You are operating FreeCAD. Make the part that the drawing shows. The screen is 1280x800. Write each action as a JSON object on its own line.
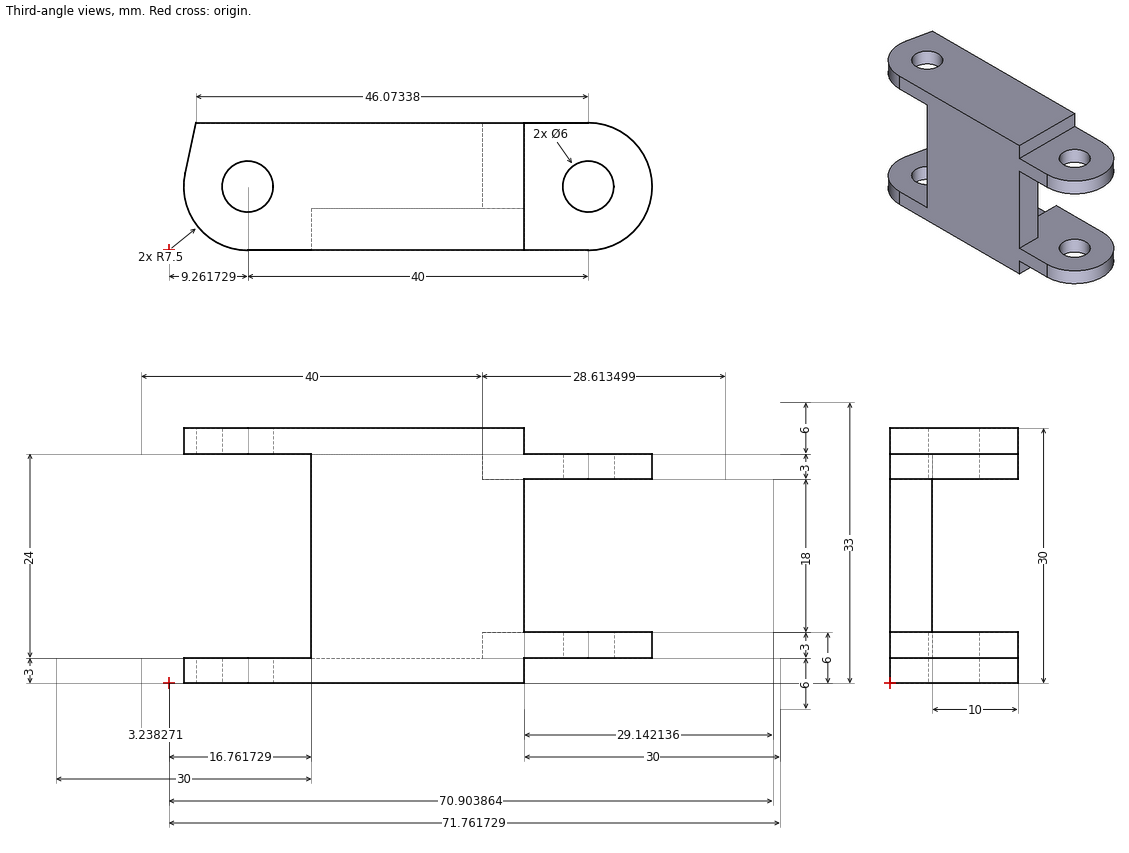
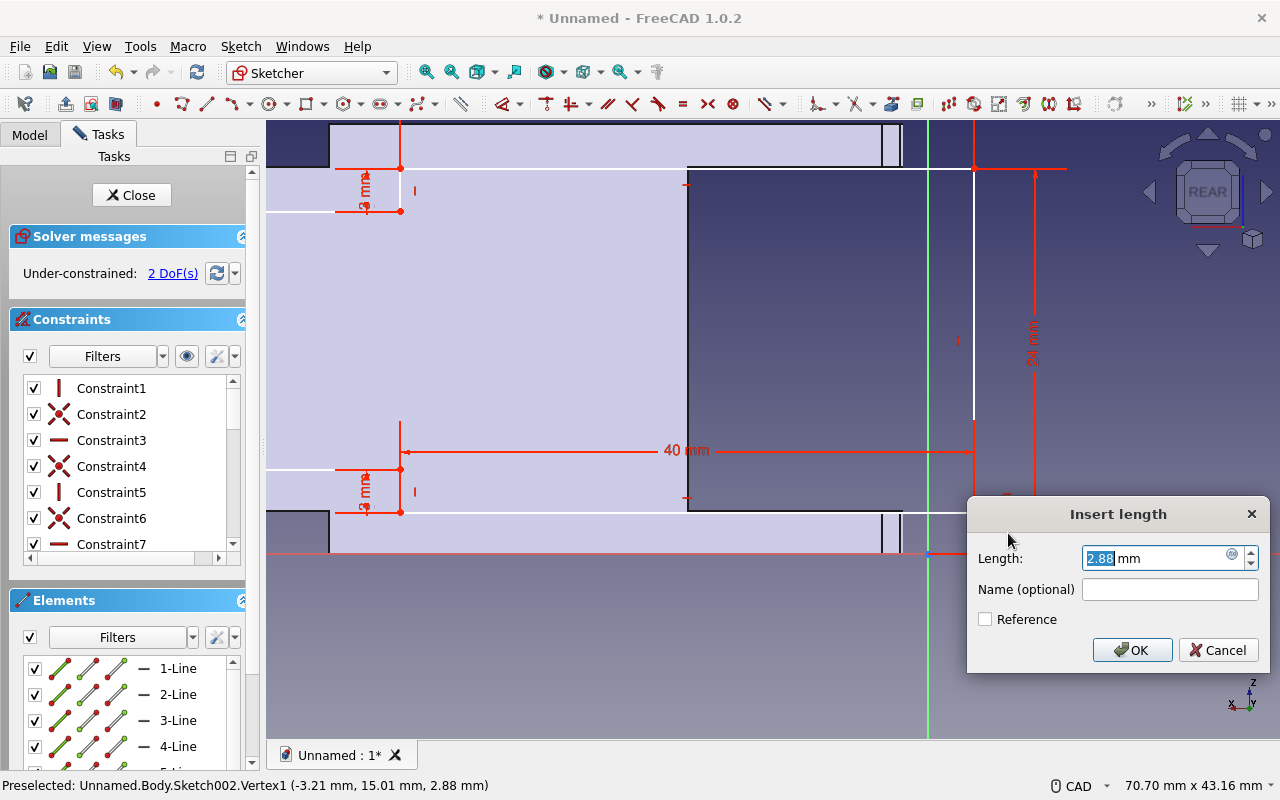
{"action": "type", "text": "3"}
{"action": "key", "text": "Return"}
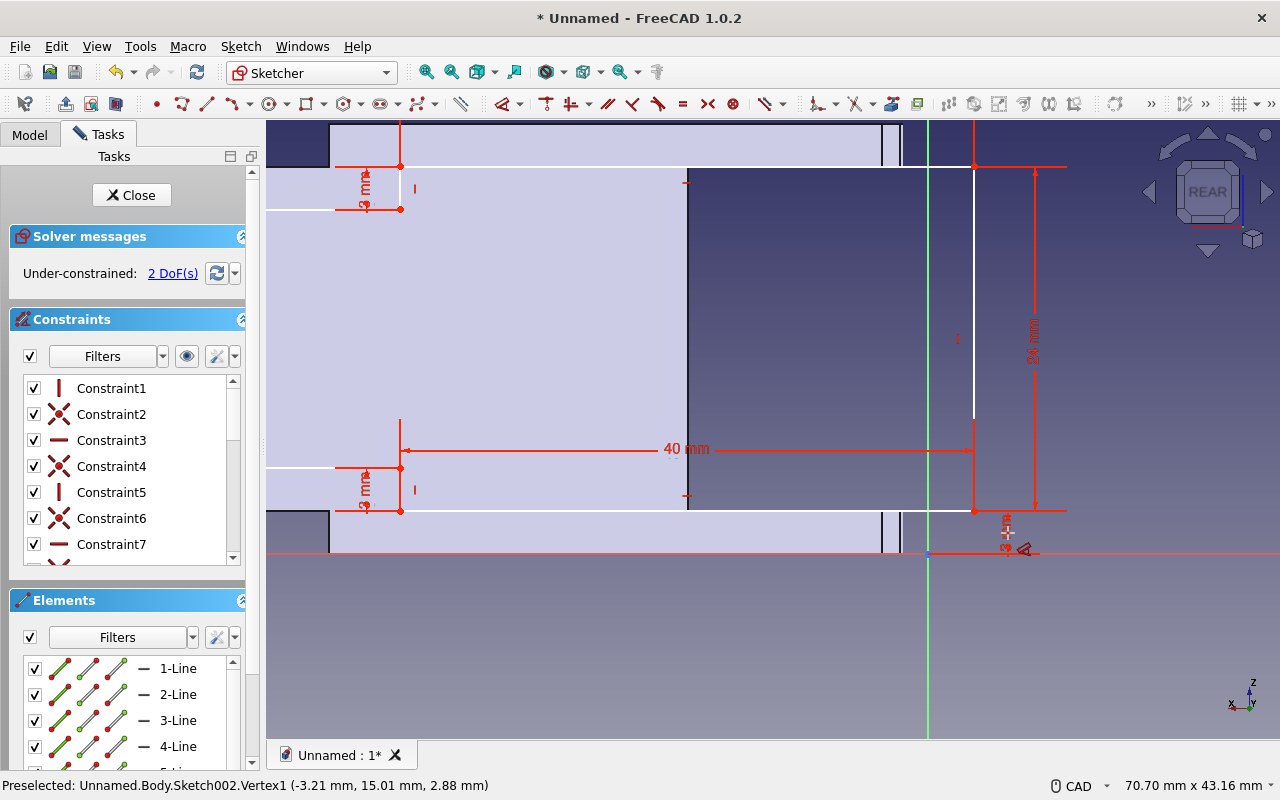
{"action": "left_click", "coordinate": [319, 210]}
{"action": "left_click", "coordinate": [347, 244]}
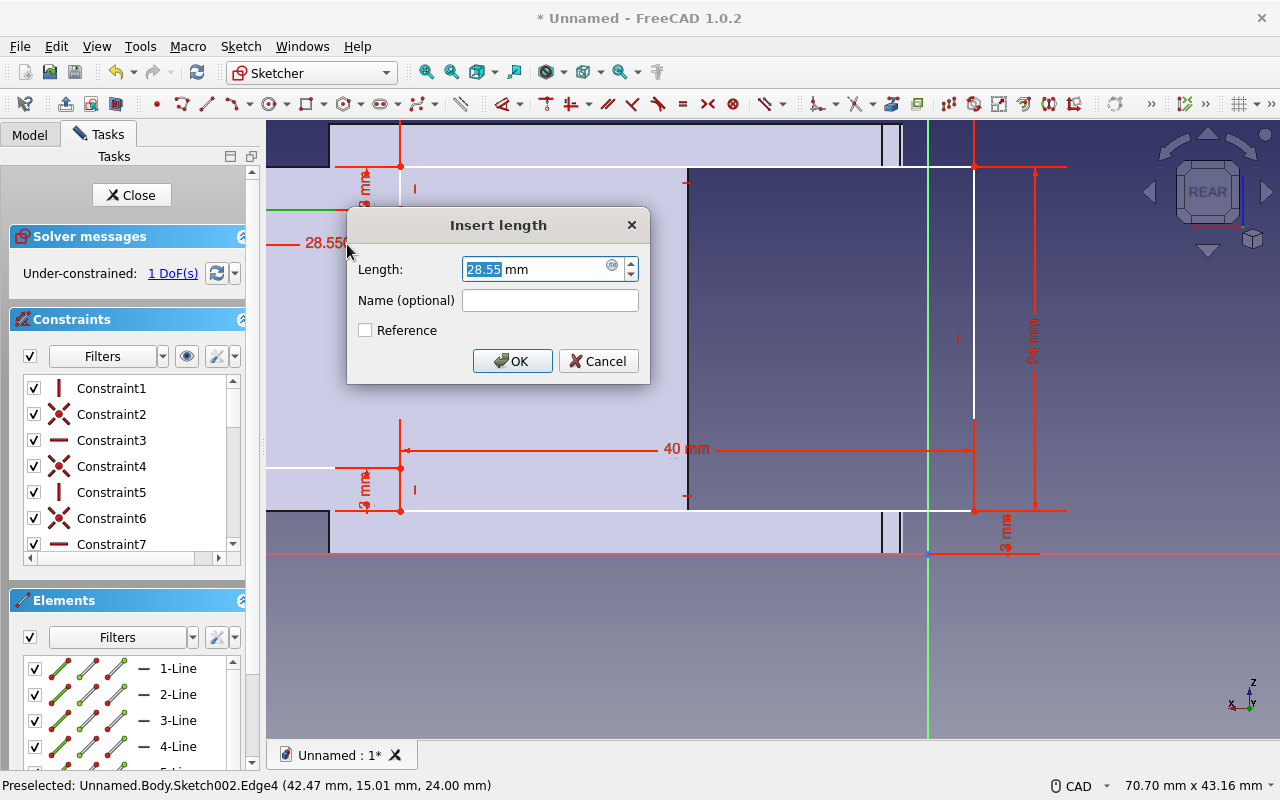
{"action": "type", "text": "28.613499"}
{"action": "key", "text": "Return"}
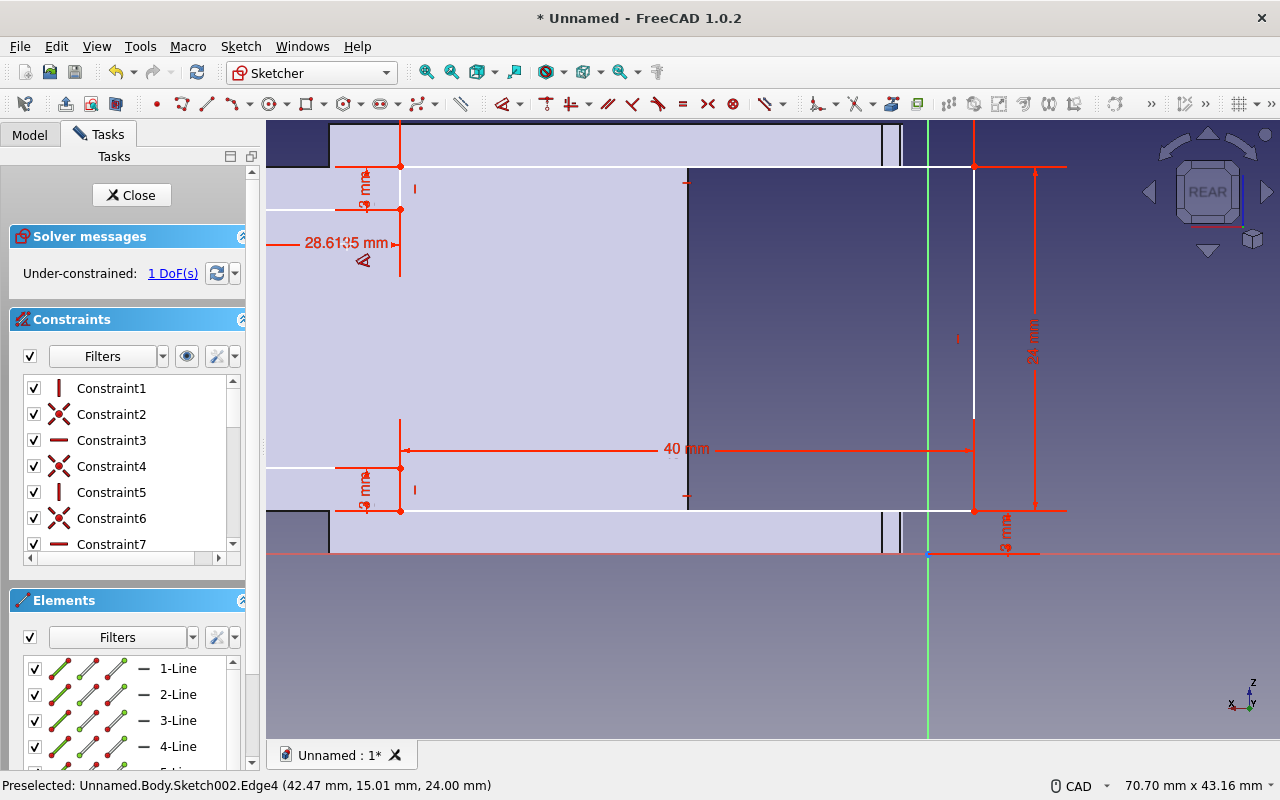
{"action": "left_click", "coordinate": [974, 511]}
{"action": "left_click", "coordinate": [951, 588]}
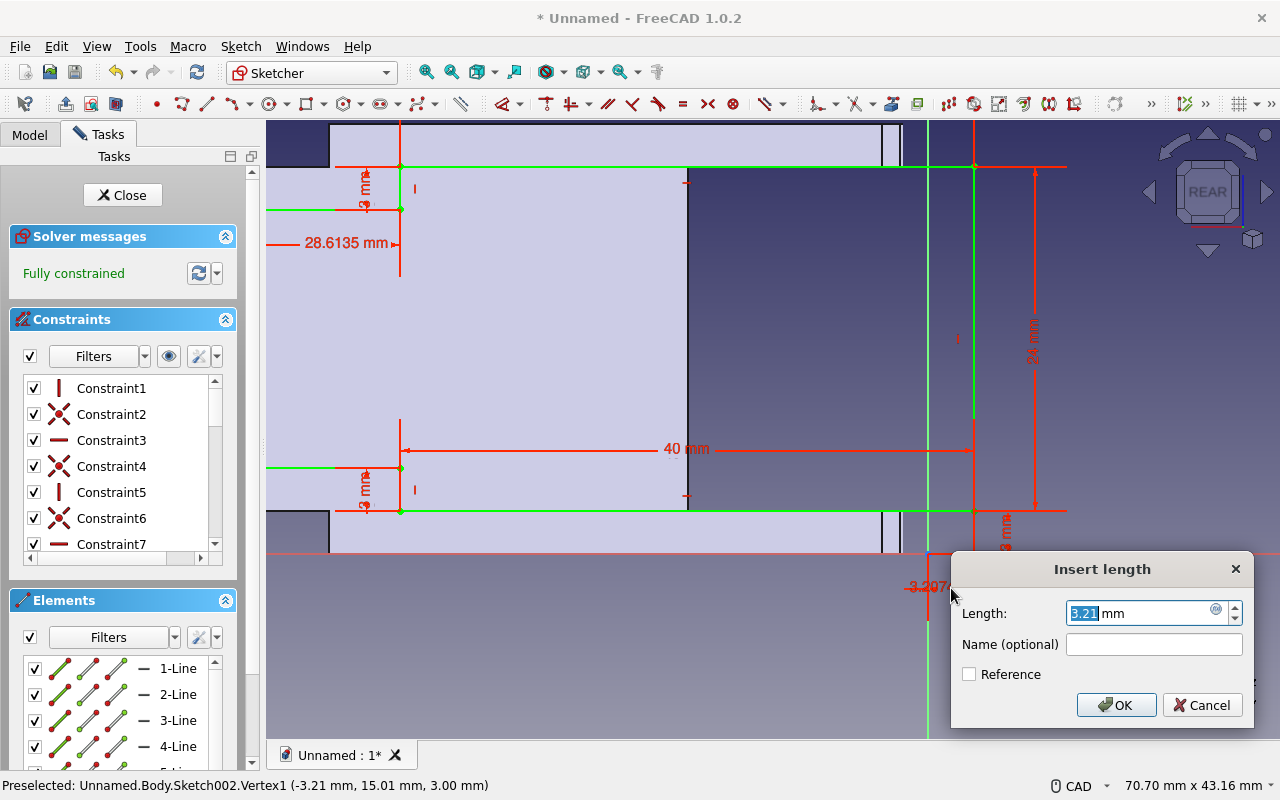
{"action": "type", "text": "3.238271"}
{"action": "key", "text": "Return"}
{"action": "key", "text": "Escape"}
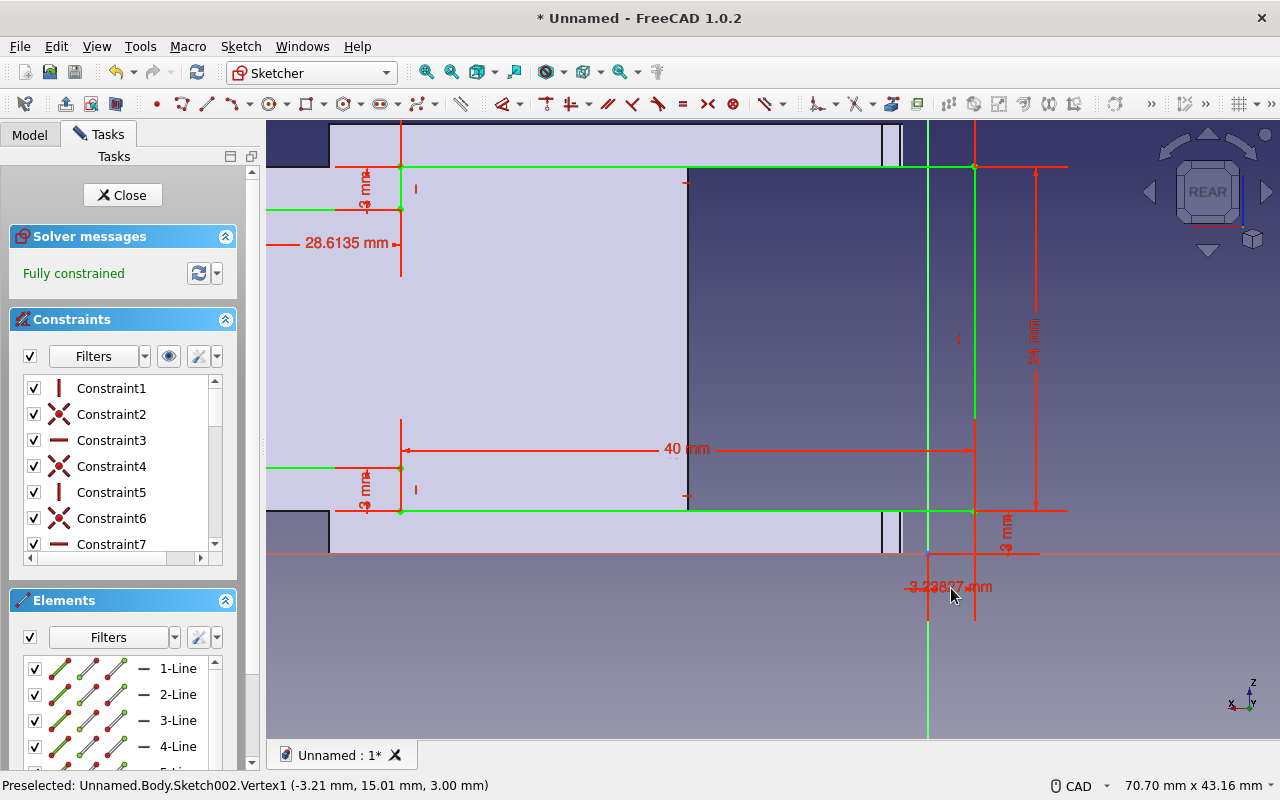
{"action": "left_click", "coordinate": [123, 195]}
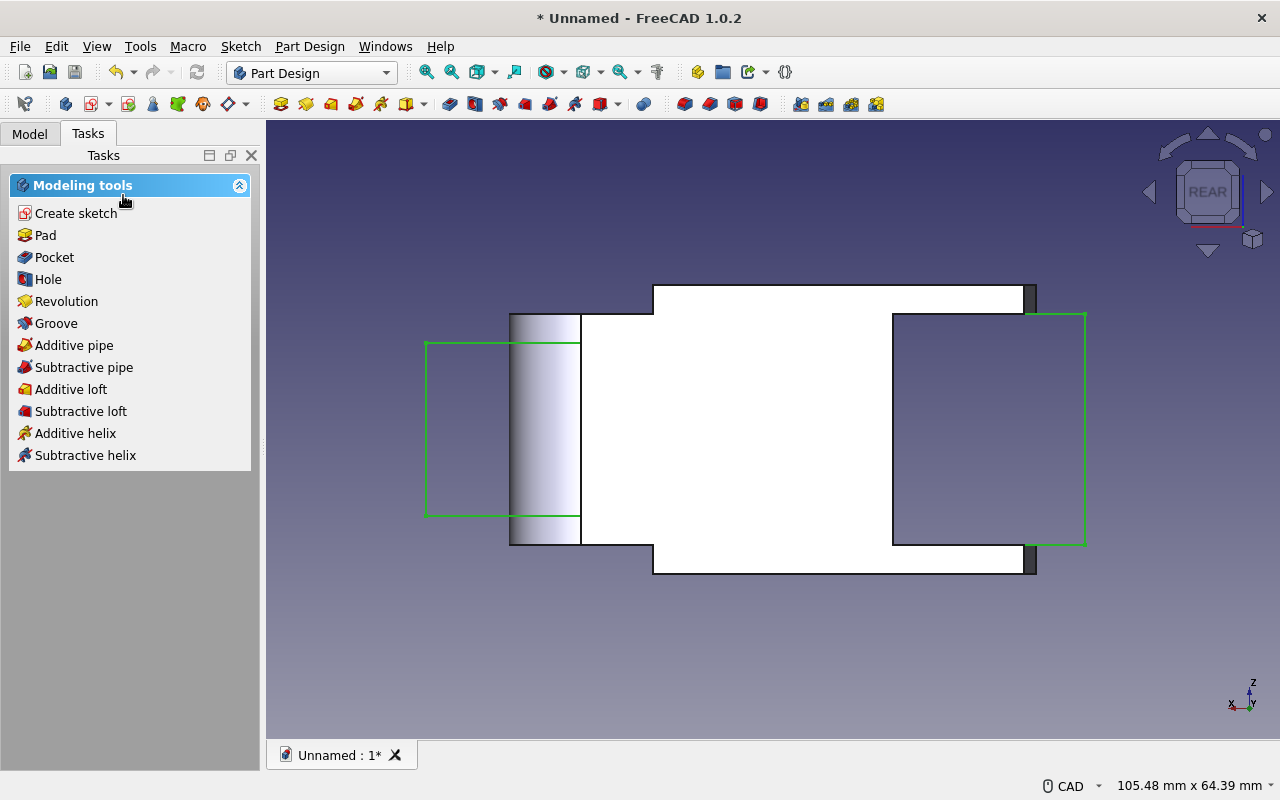
{"action": "left_click", "coordinate": [450, 104]}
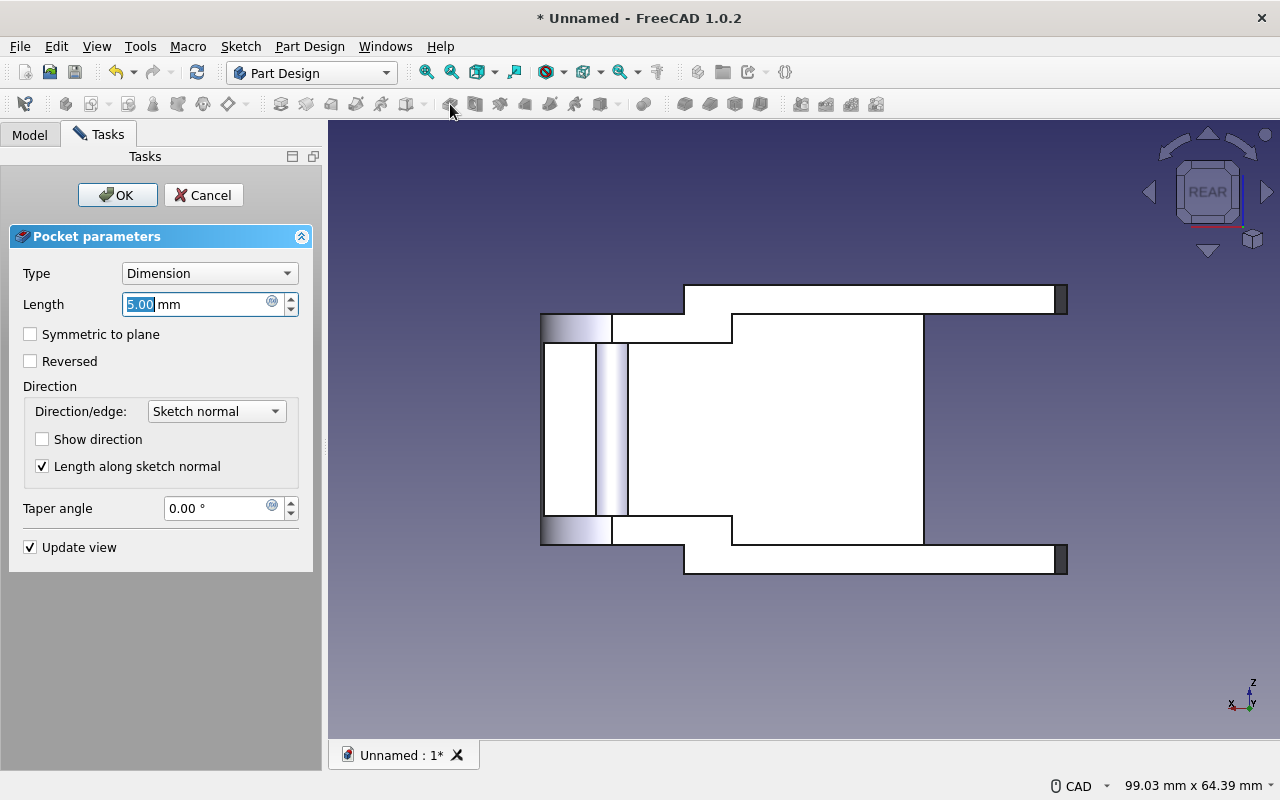
{"action": "type", "text": "10"}
{"action": "key", "text": "Tab"}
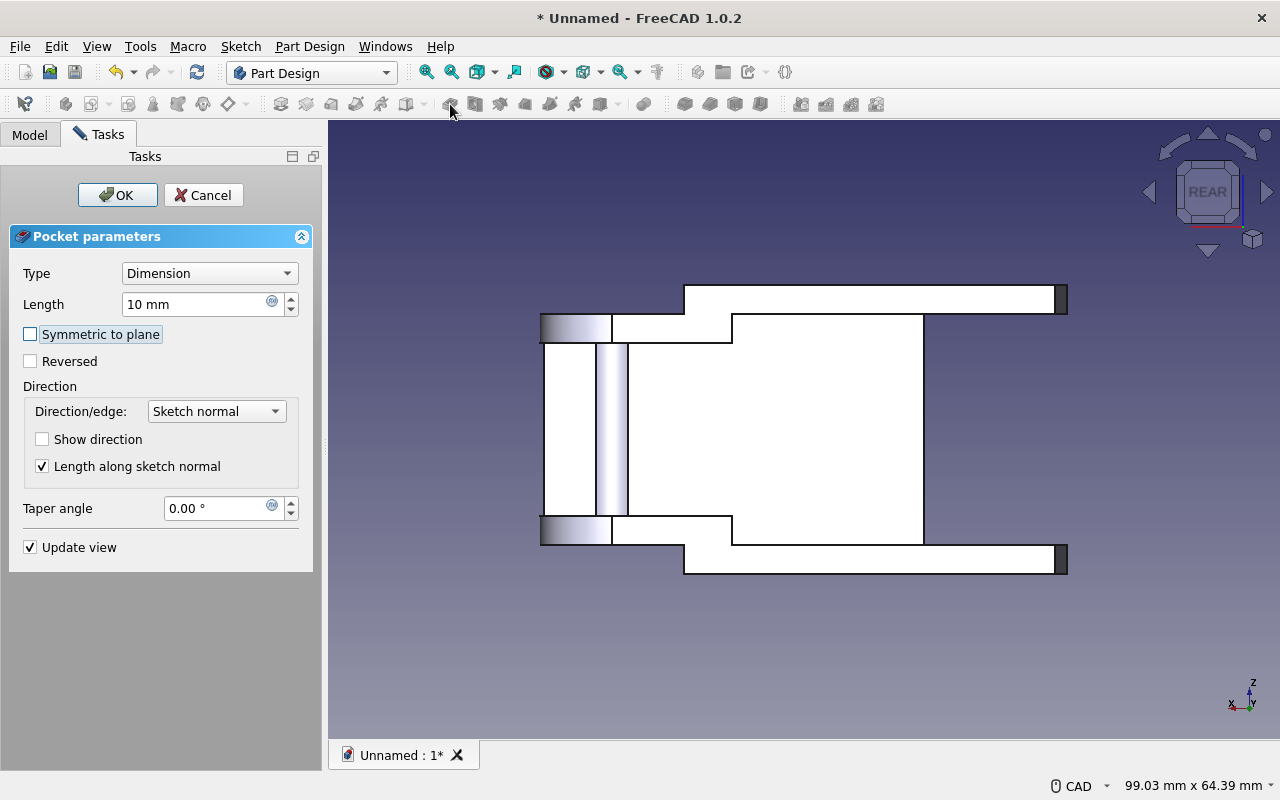
{"action": "left_click", "coordinate": [118, 195]}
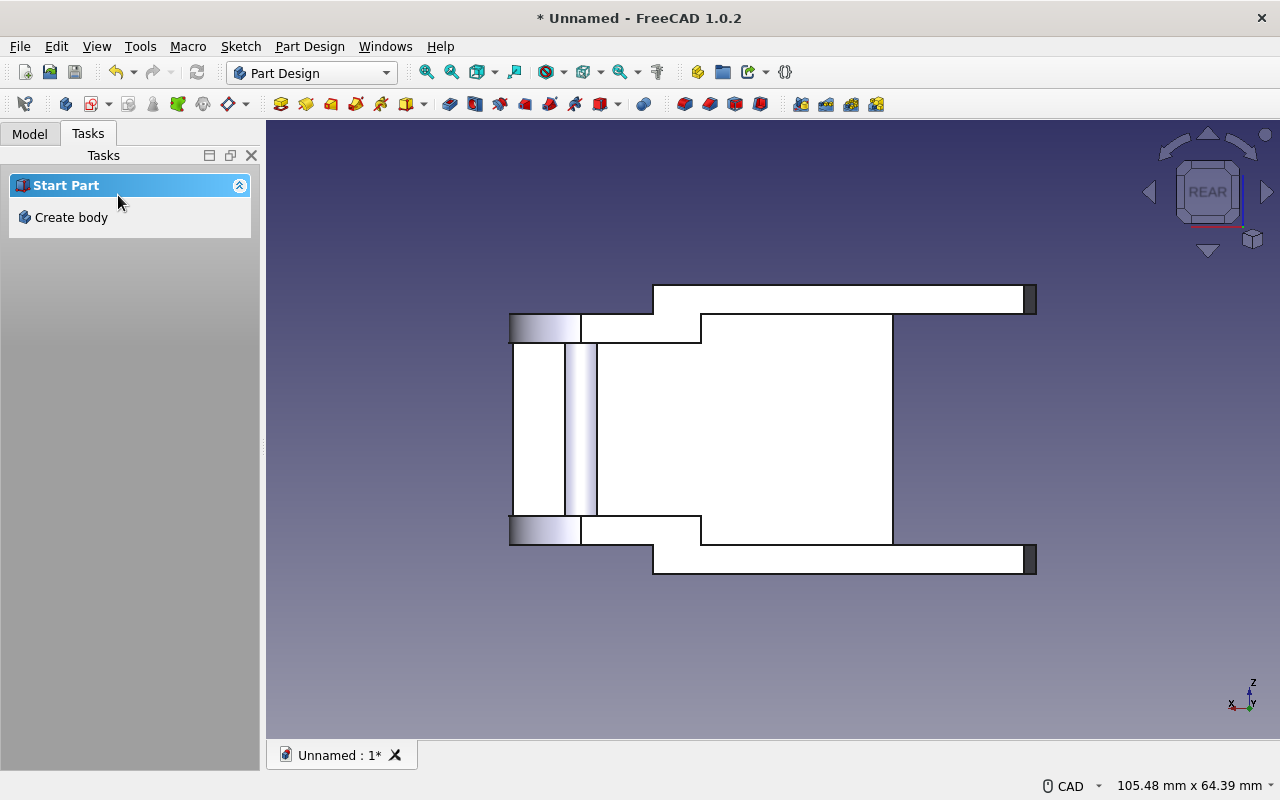
{"action": "left_click", "coordinate": [787, 429]}